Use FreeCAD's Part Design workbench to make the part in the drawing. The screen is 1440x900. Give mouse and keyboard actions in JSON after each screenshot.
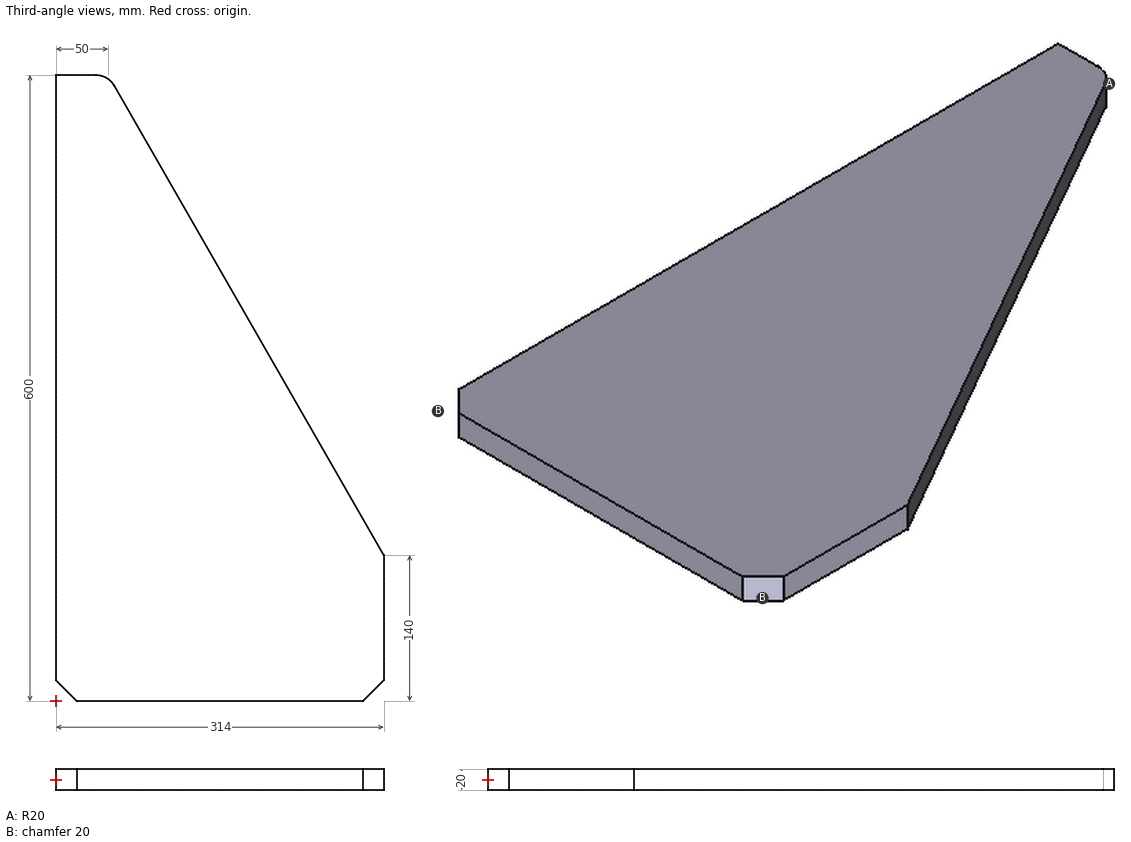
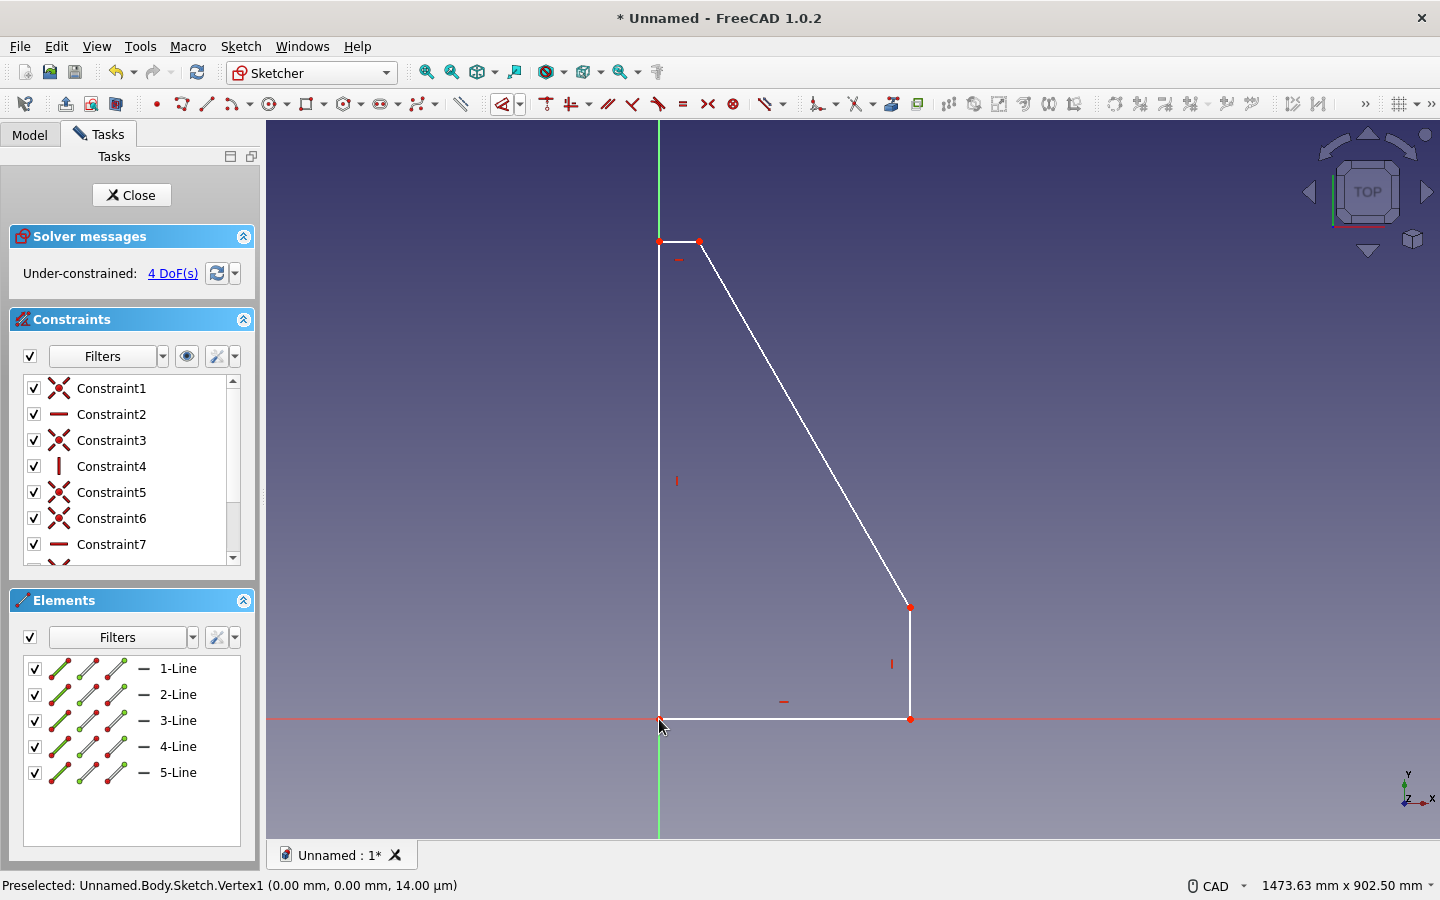
{"action": "key", "text": "d"}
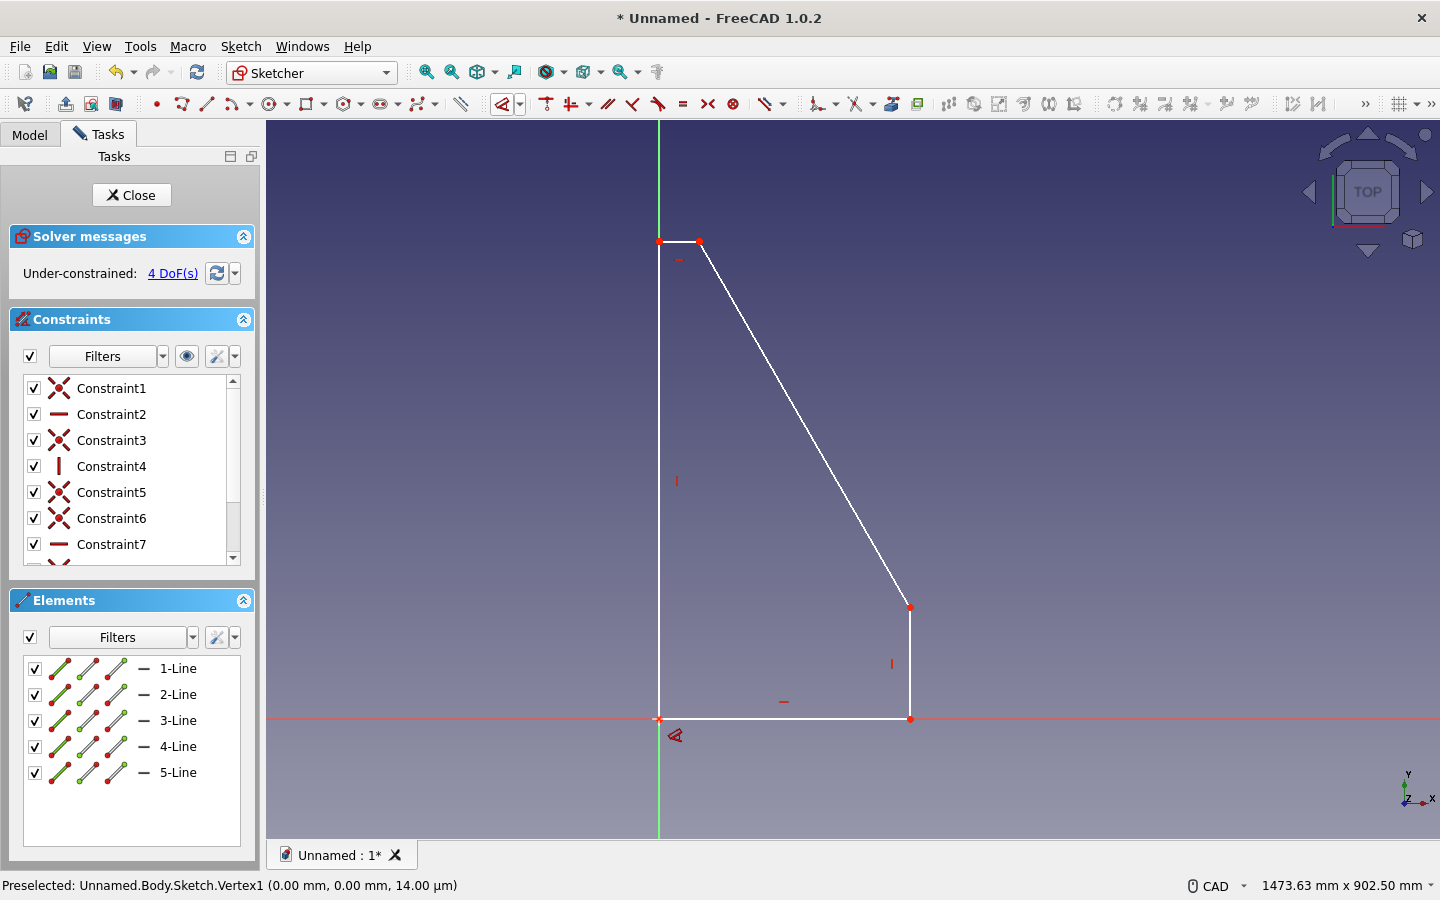
{"action": "left_click", "coordinate": [687, 242]}
{"action": "left_click", "coordinate": [679, 208]}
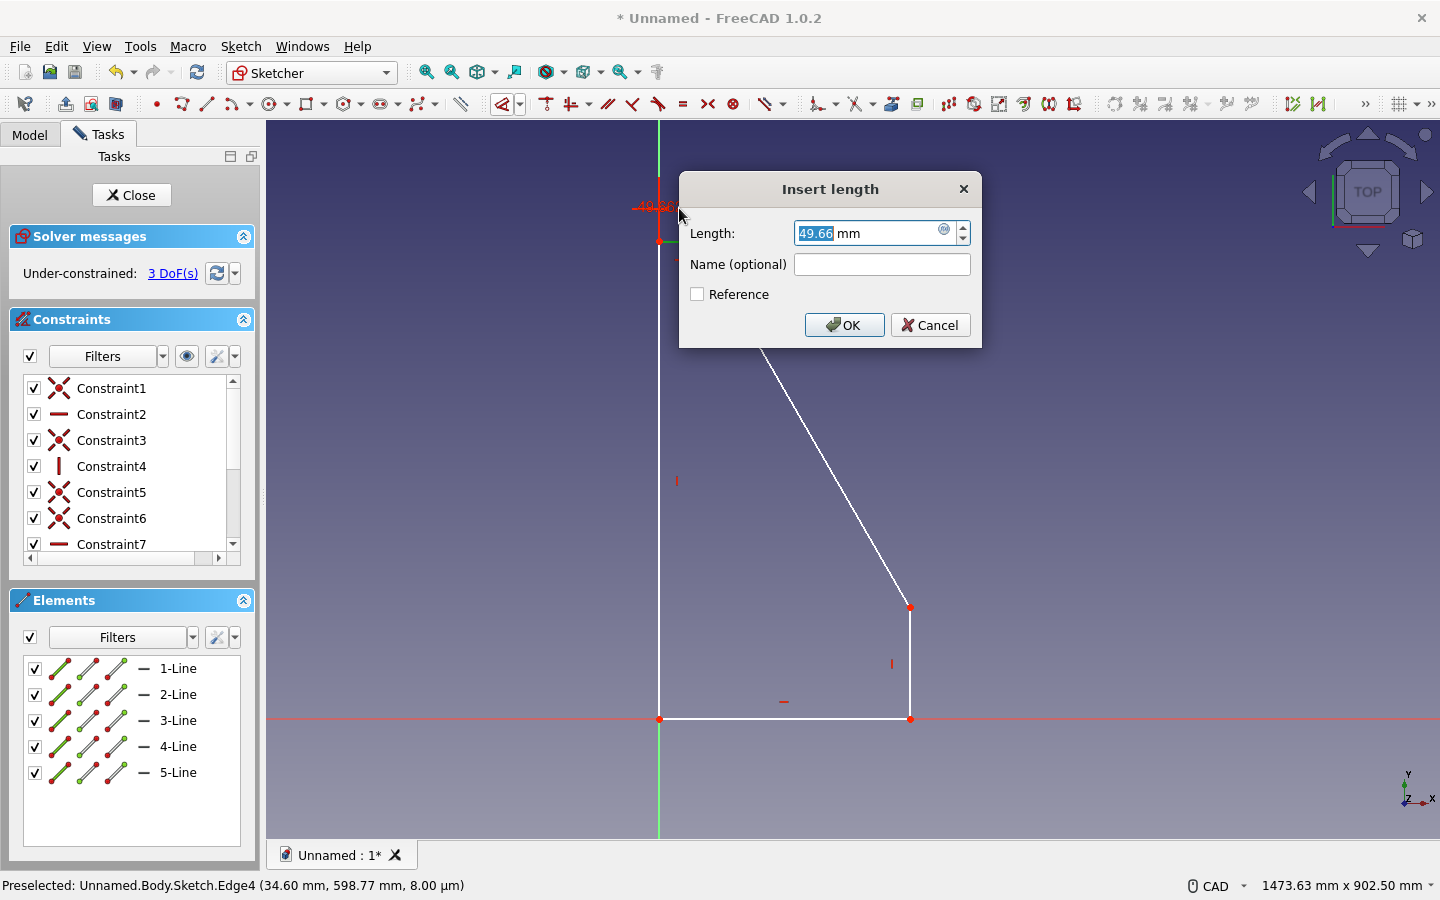
{"action": "type", "text": "50"}
{"action": "key", "text": "Return"}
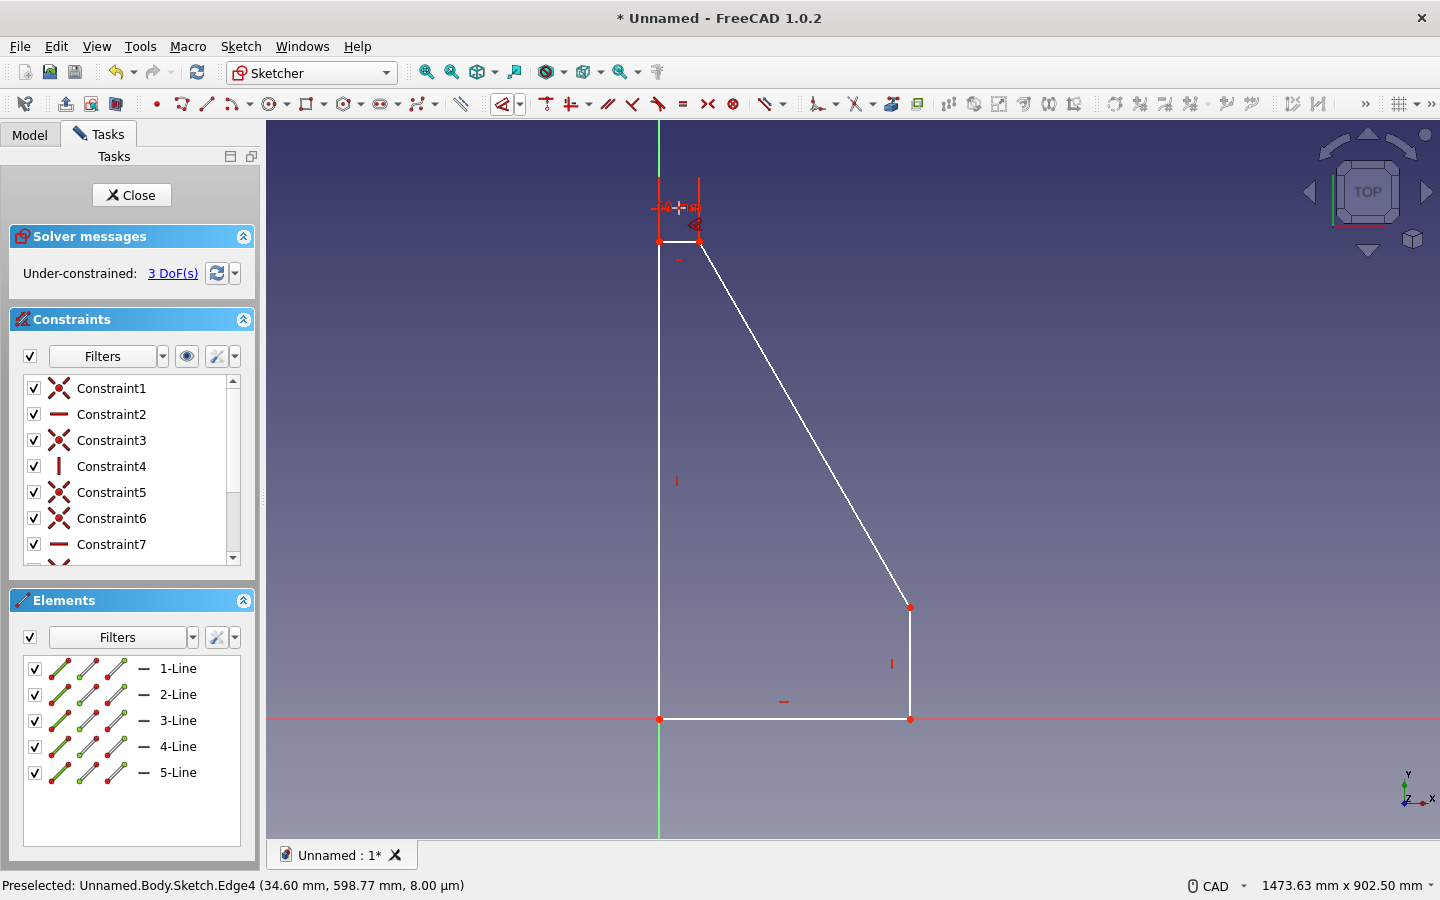
{"action": "left_click", "coordinate": [735, 719]}
{"action": "left_click", "coordinate": [785, 753]}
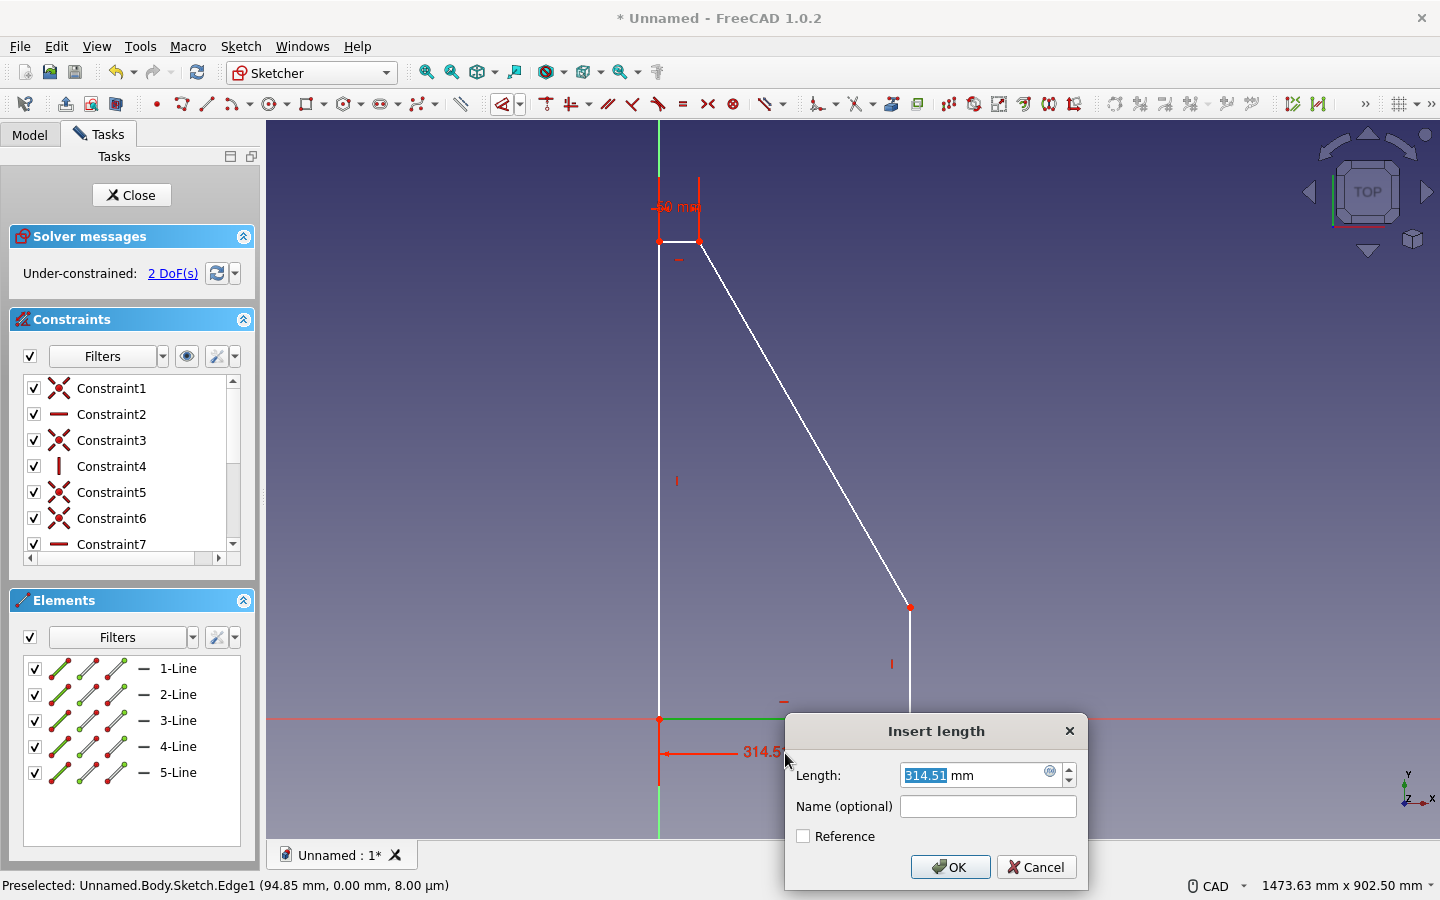
{"action": "type", "text": "314"}
{"action": "key", "text": "Return"}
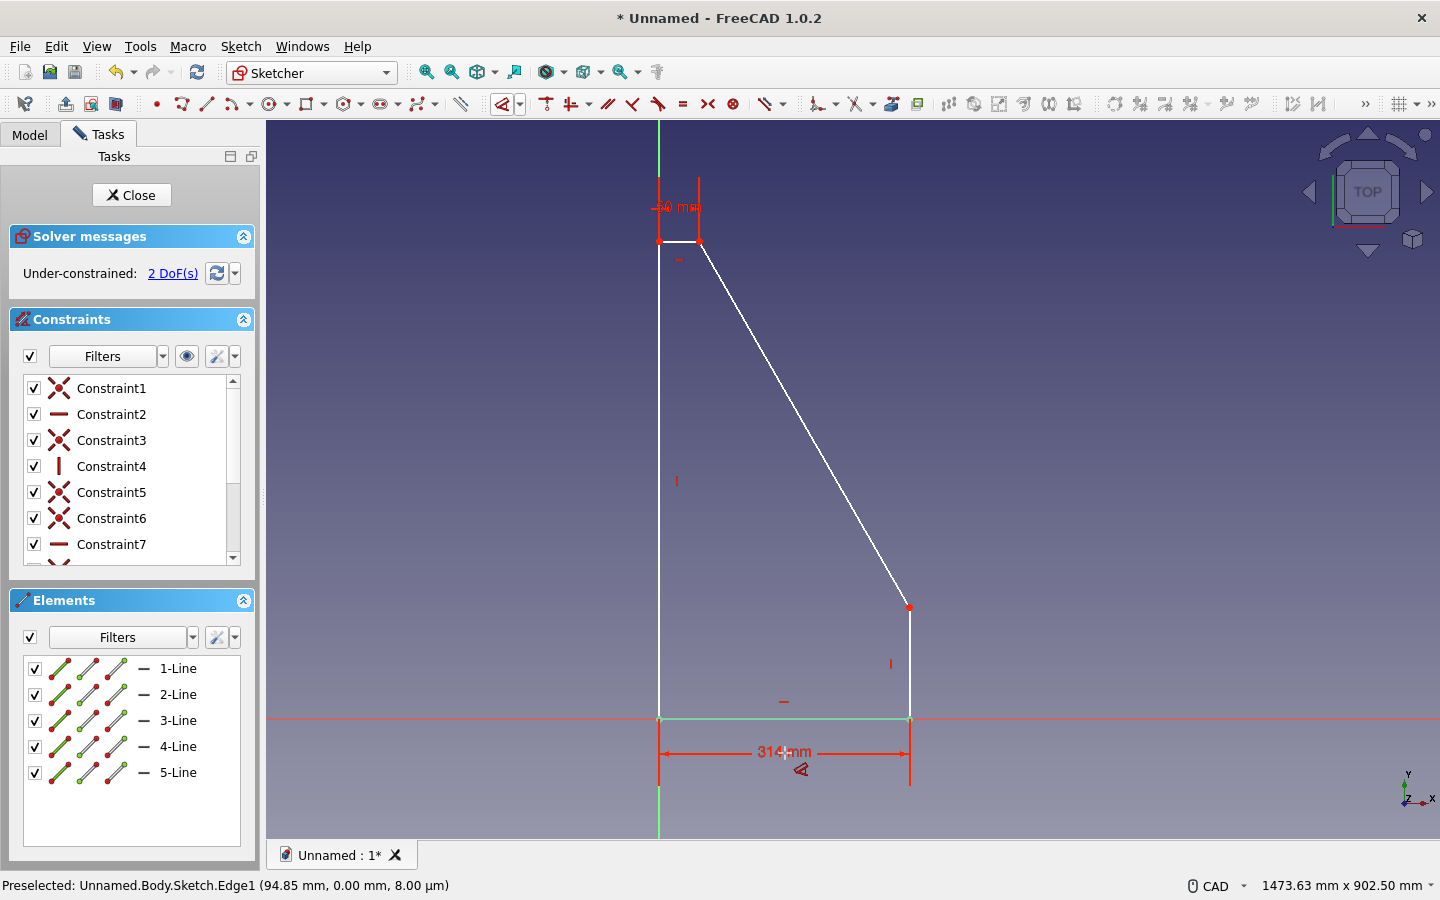
{"action": "left_click", "coordinate": [910, 686]}
{"action": "left_click", "coordinate": [944, 664]}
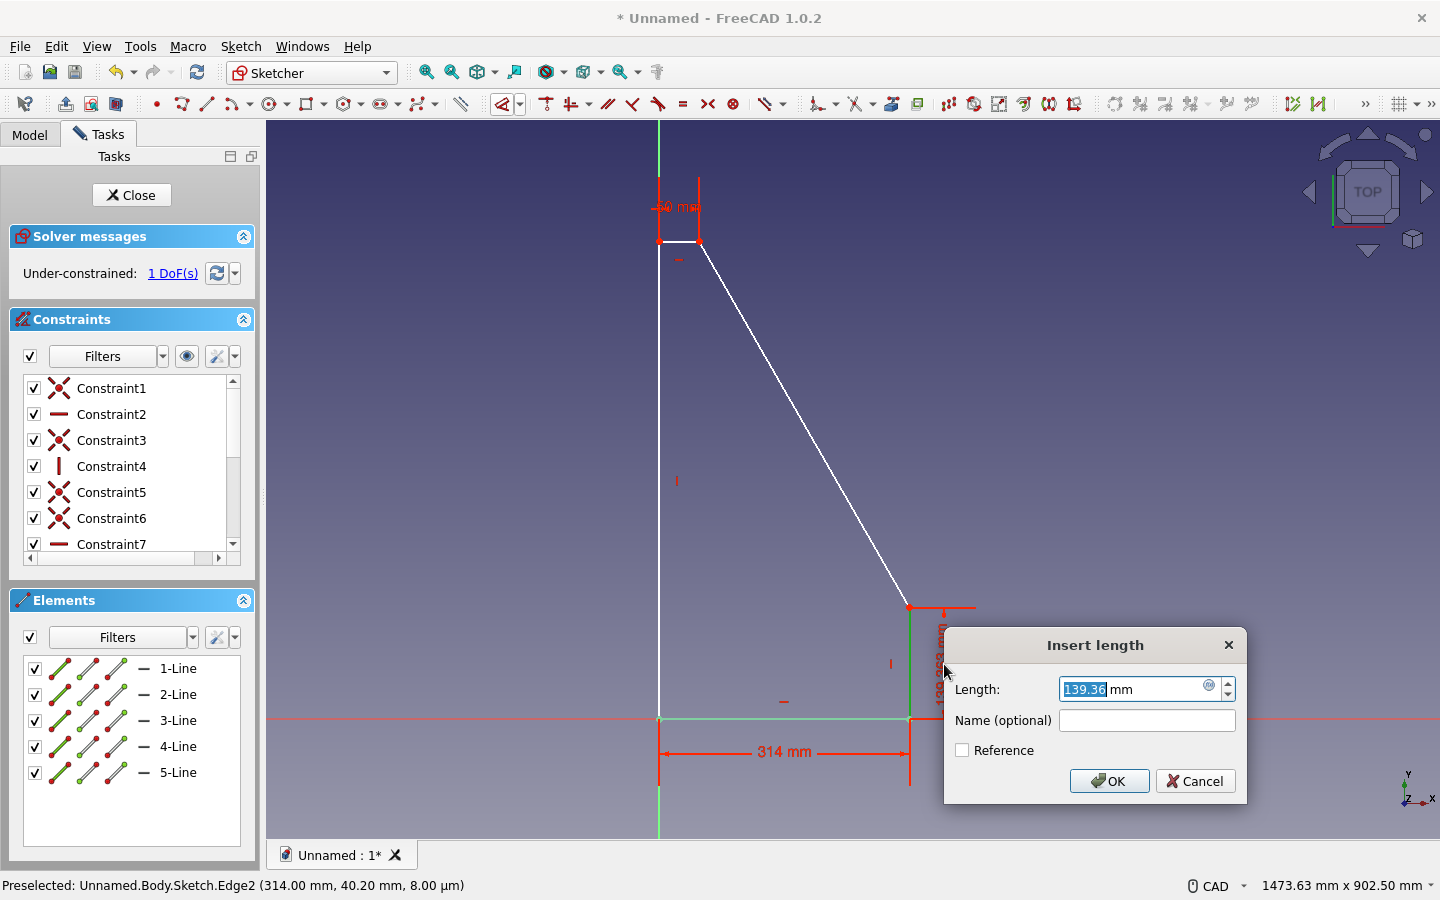
{"action": "type", "text": "140"}
{"action": "key", "text": "Return"}